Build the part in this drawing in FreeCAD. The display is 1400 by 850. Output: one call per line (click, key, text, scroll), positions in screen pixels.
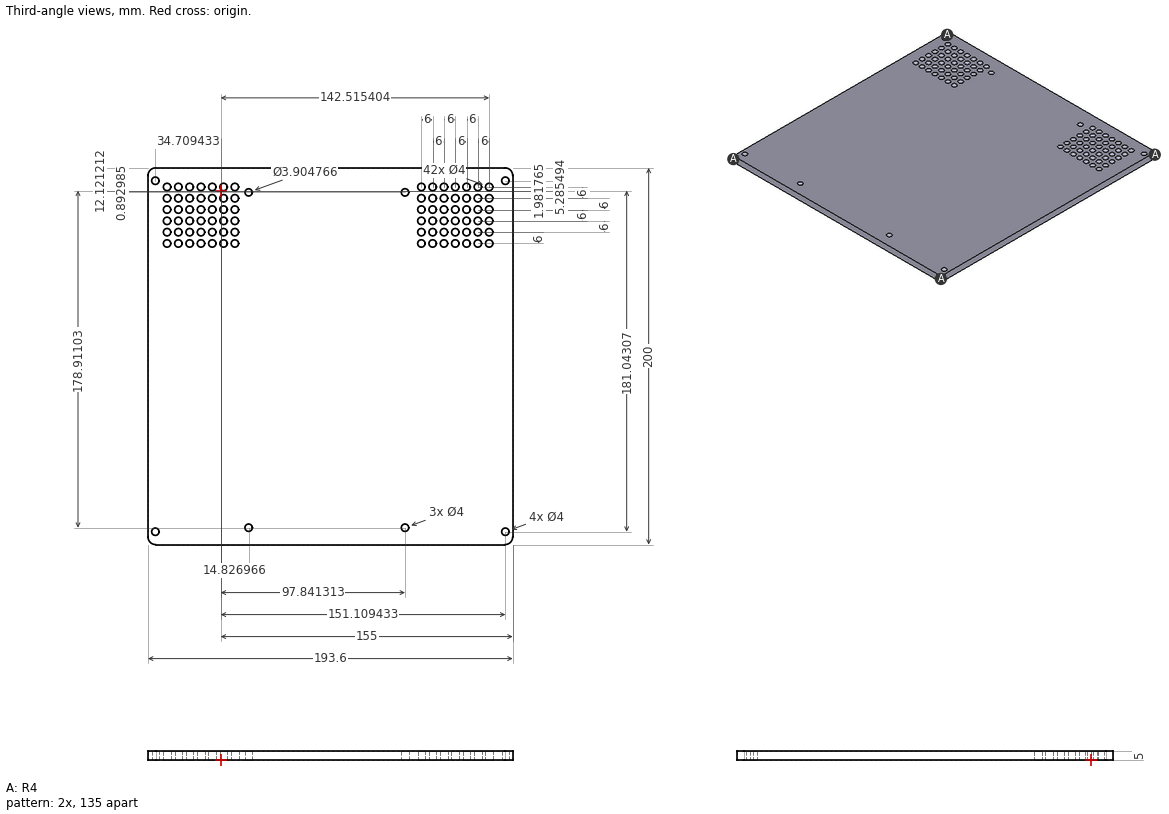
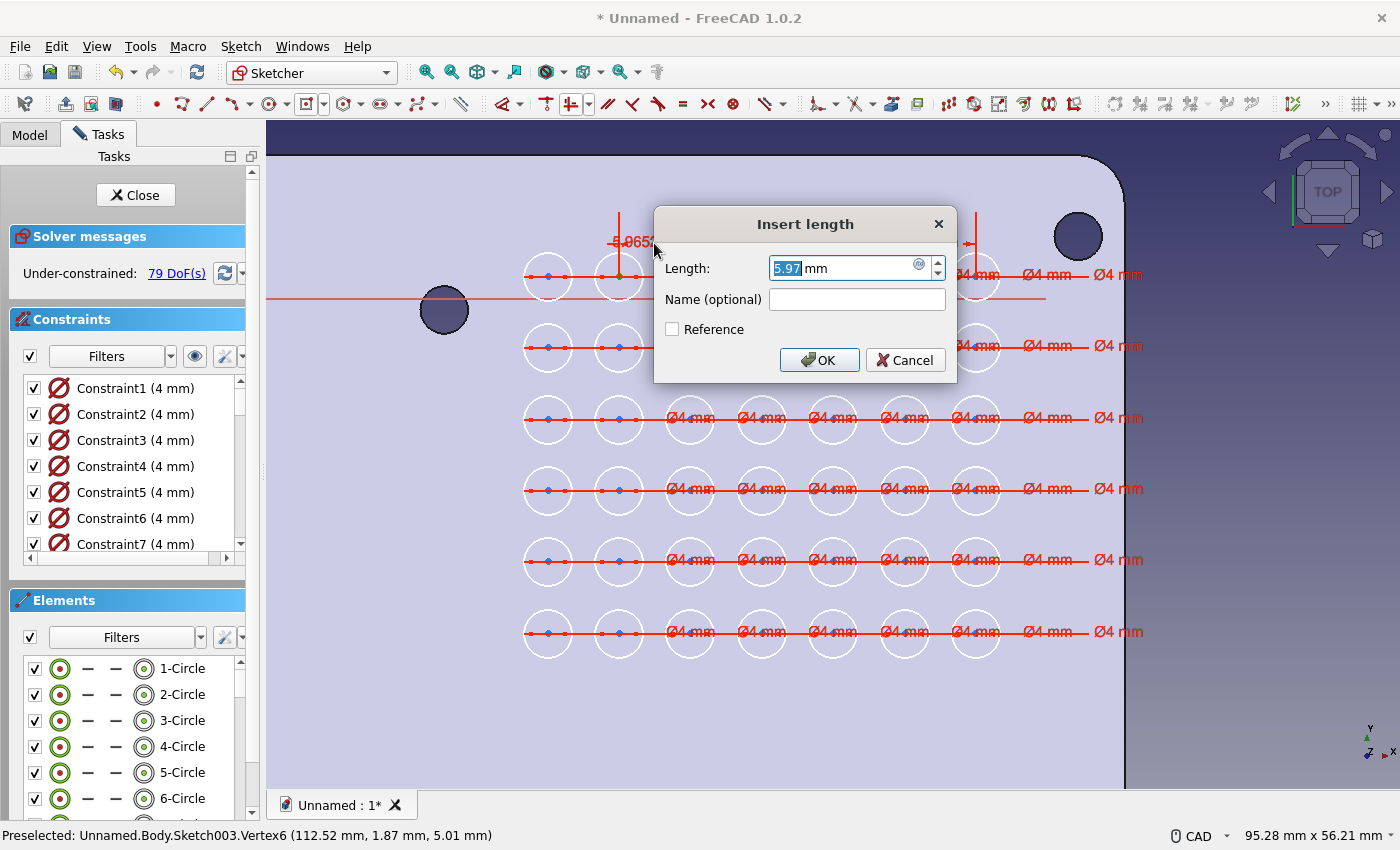
text(6)
key(Return)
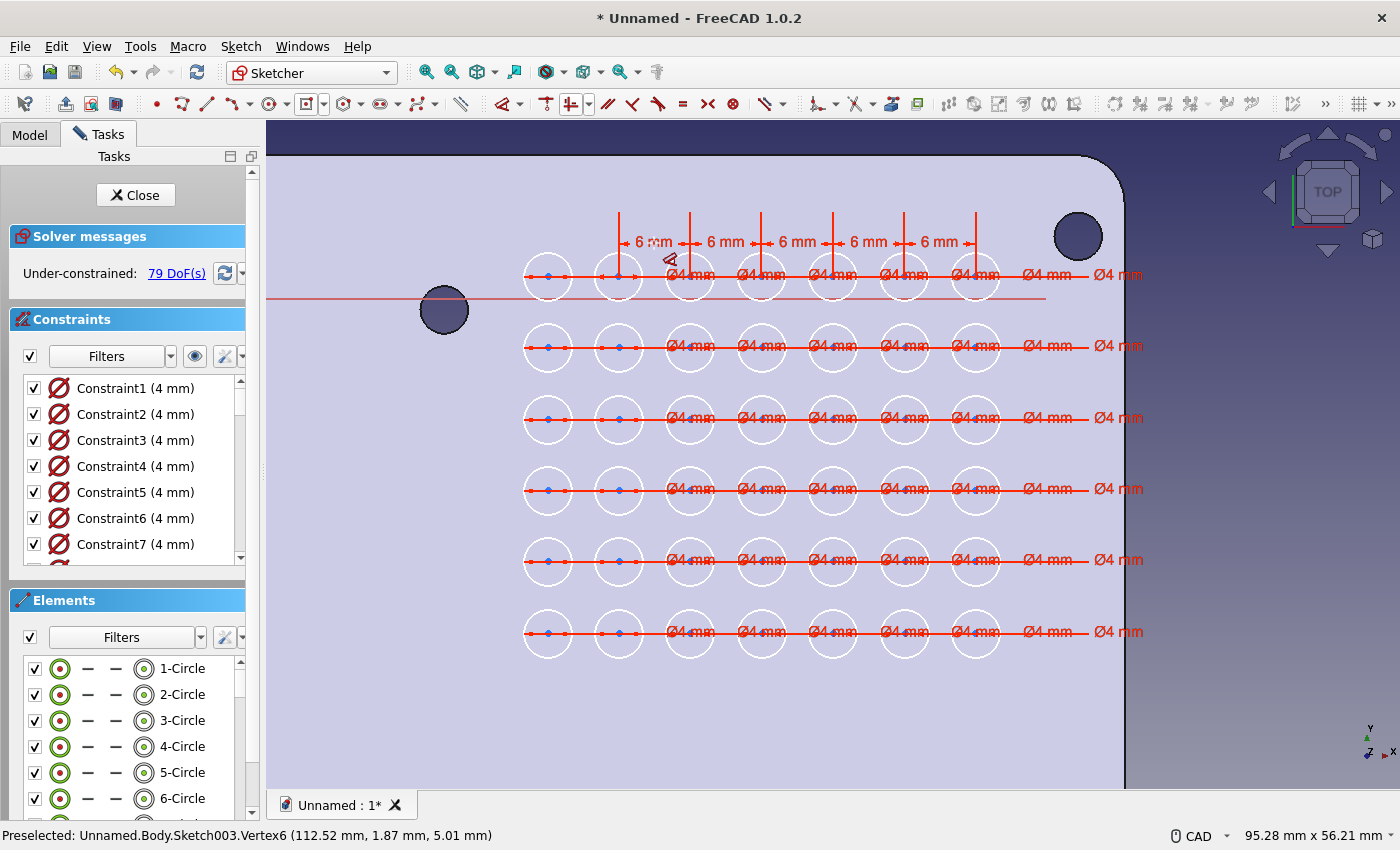
click(619, 277)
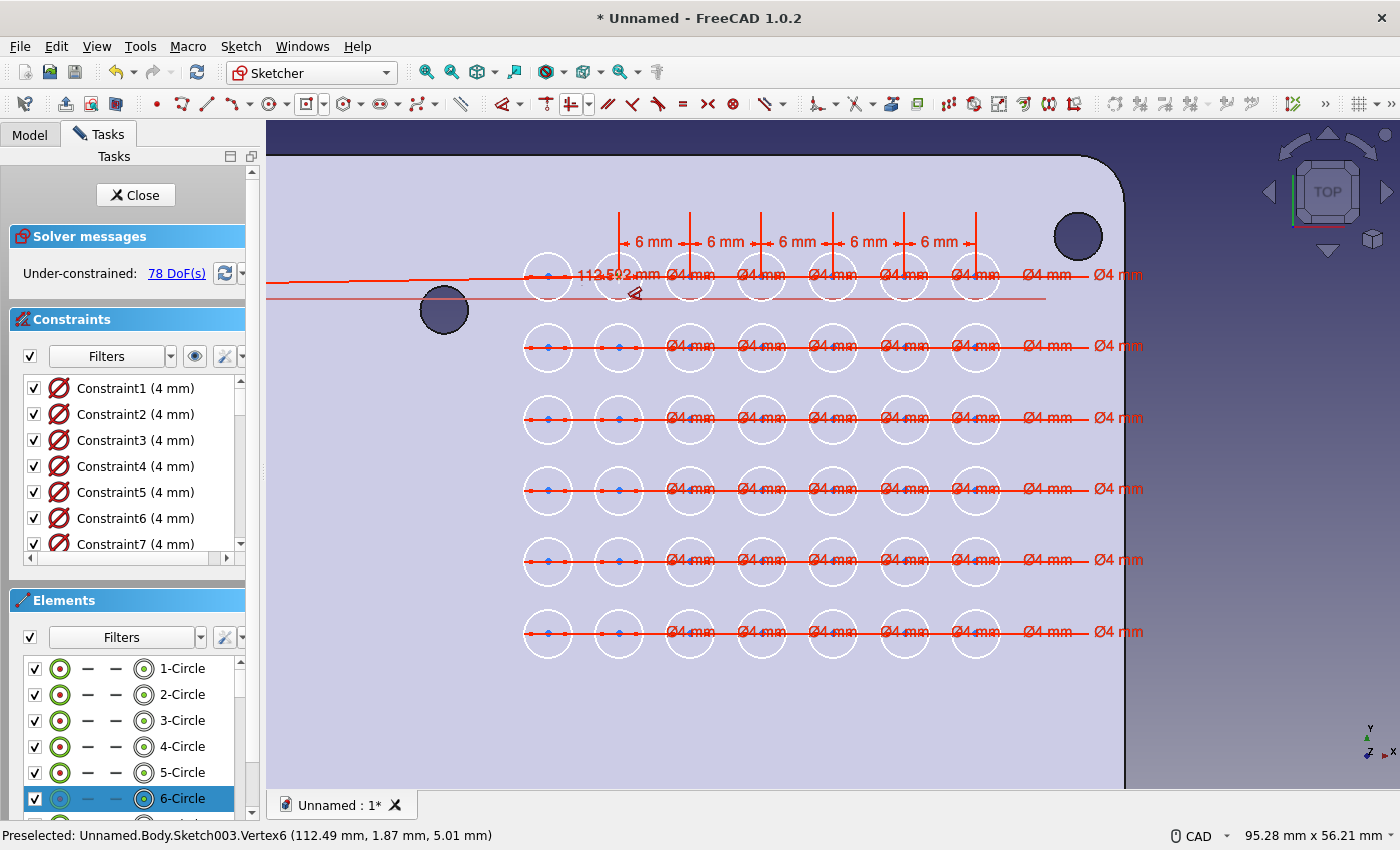
click(548, 277)
click(583, 243)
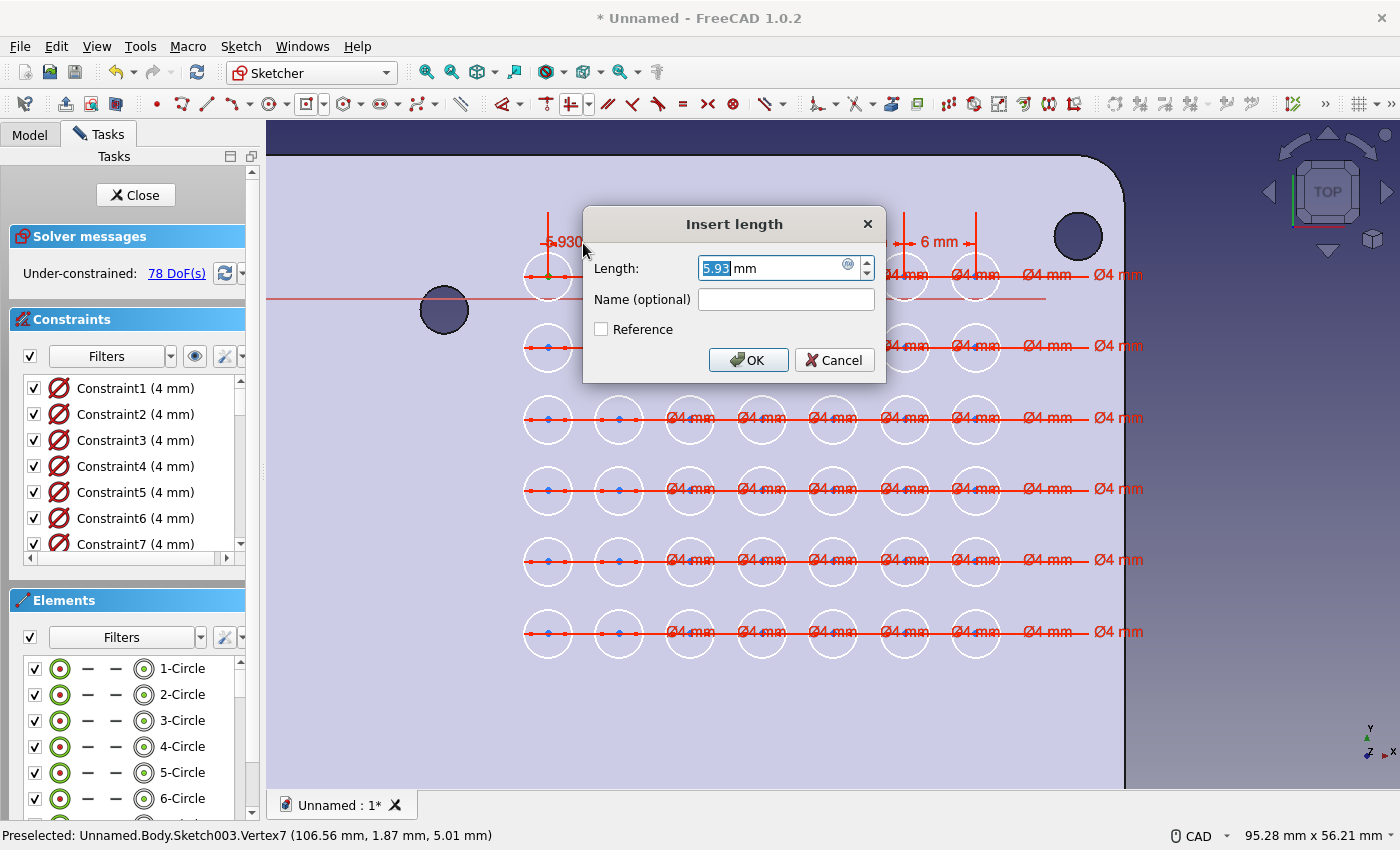
text(6)
key(Return)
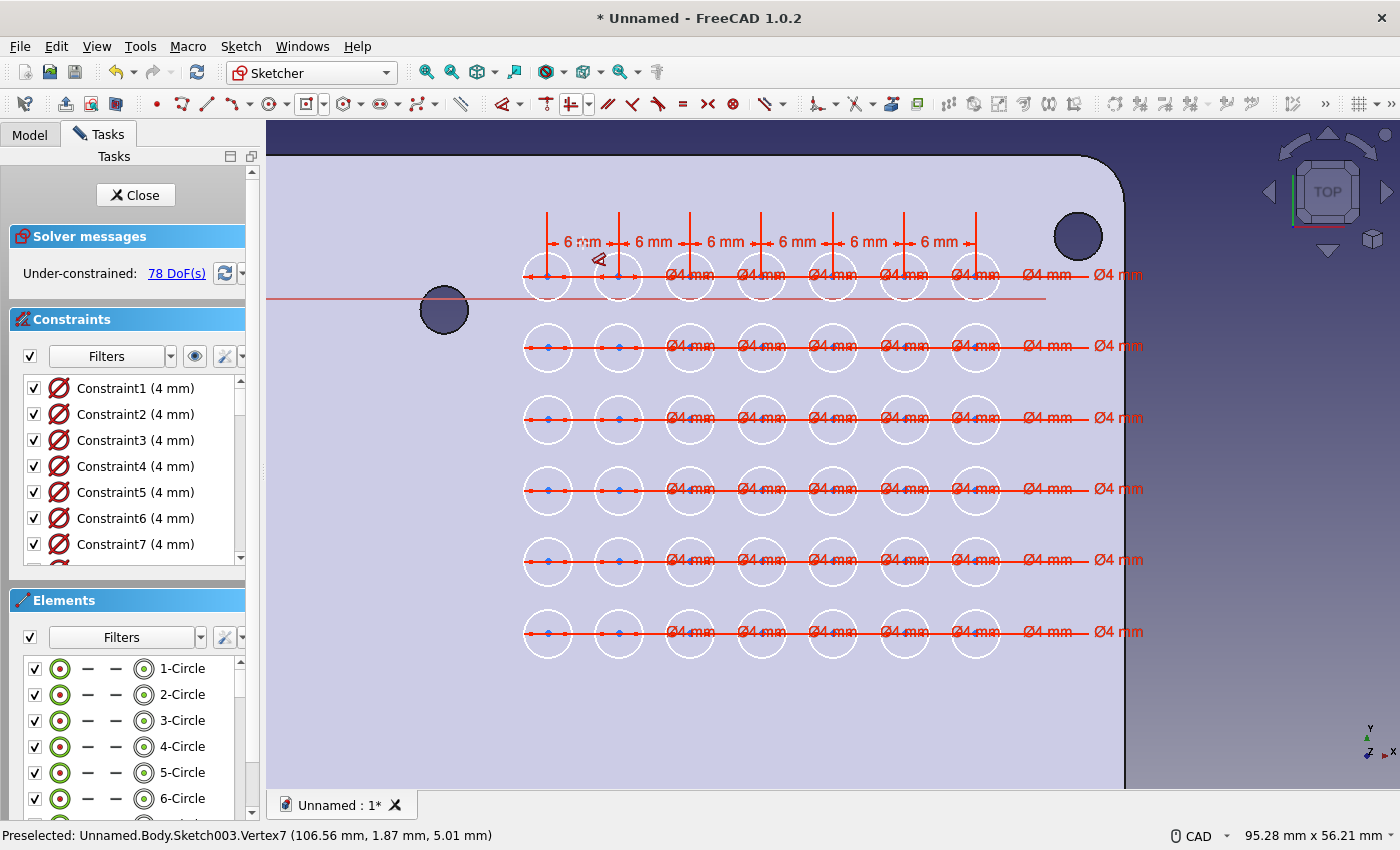
click(976, 277)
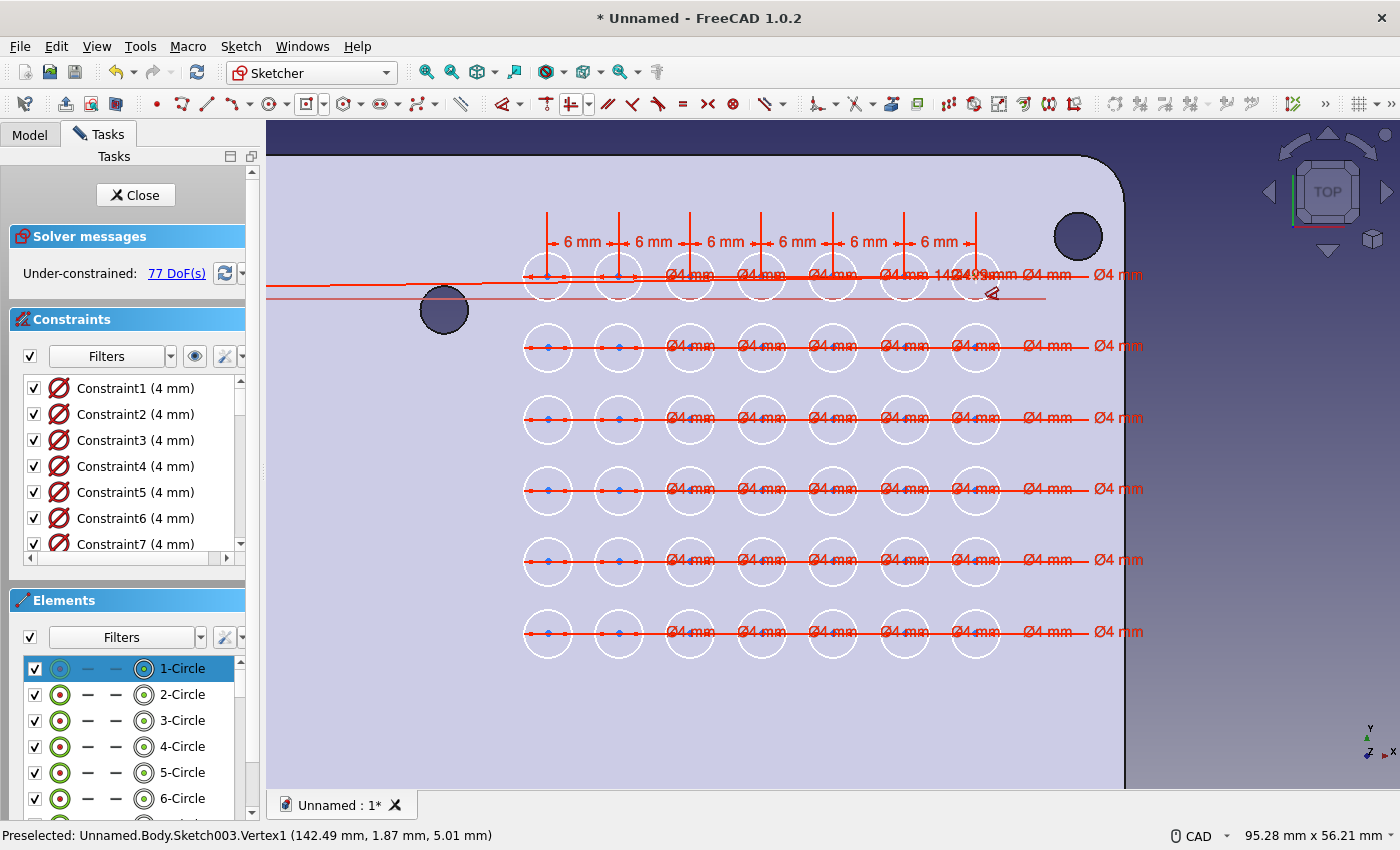
click(905, 348)
click(940, 382)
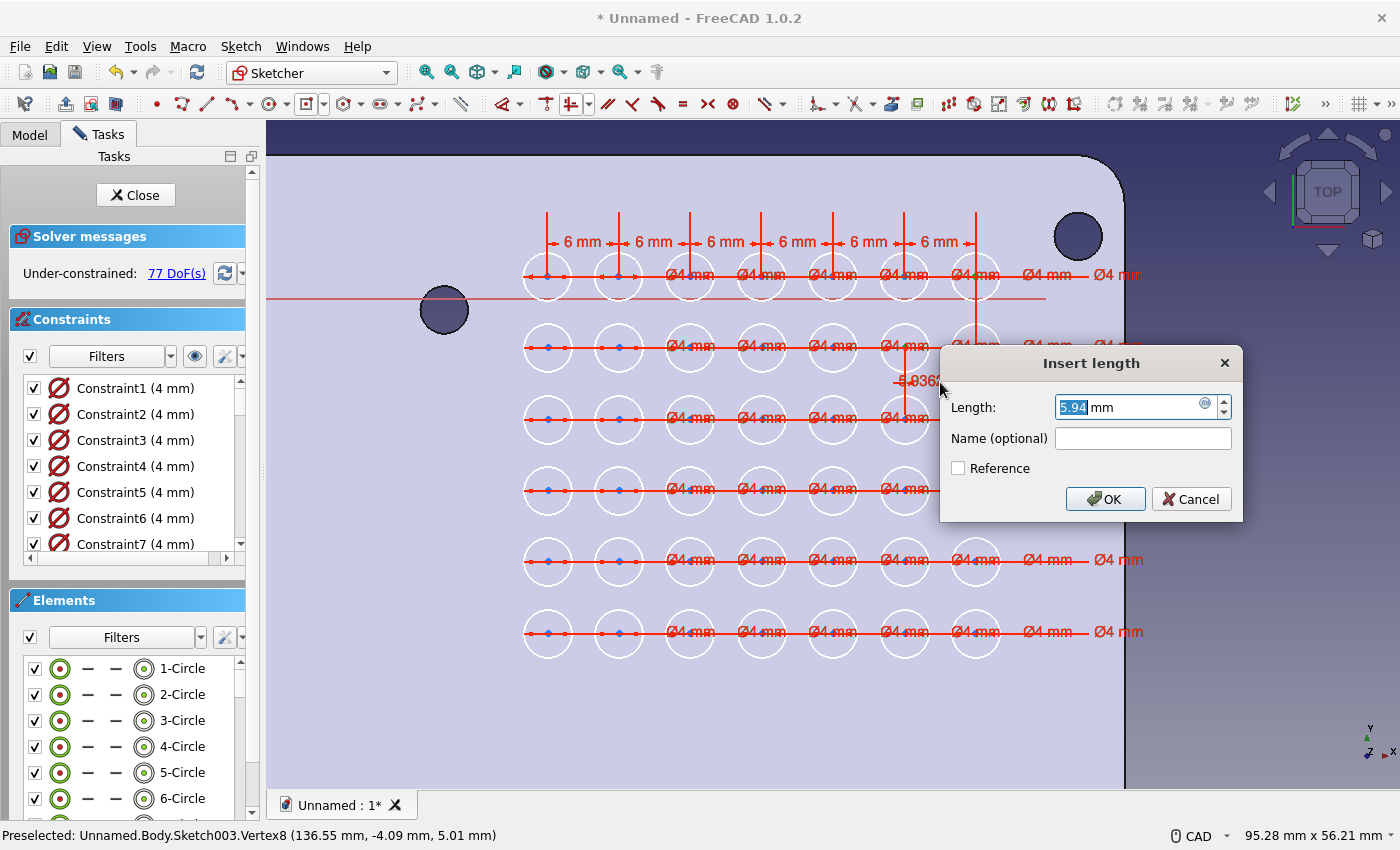
text(6)
key(Return)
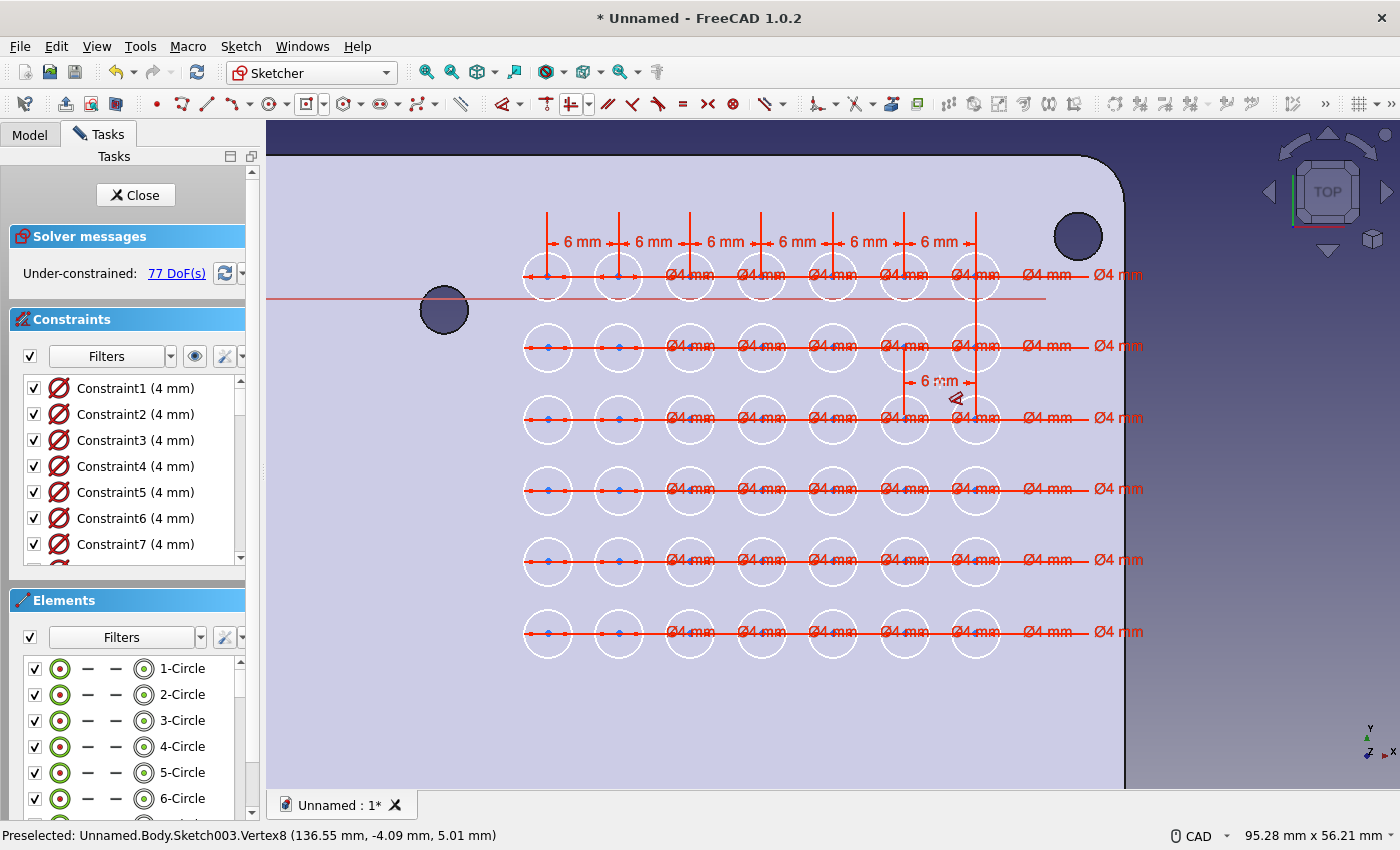
click(904, 277)